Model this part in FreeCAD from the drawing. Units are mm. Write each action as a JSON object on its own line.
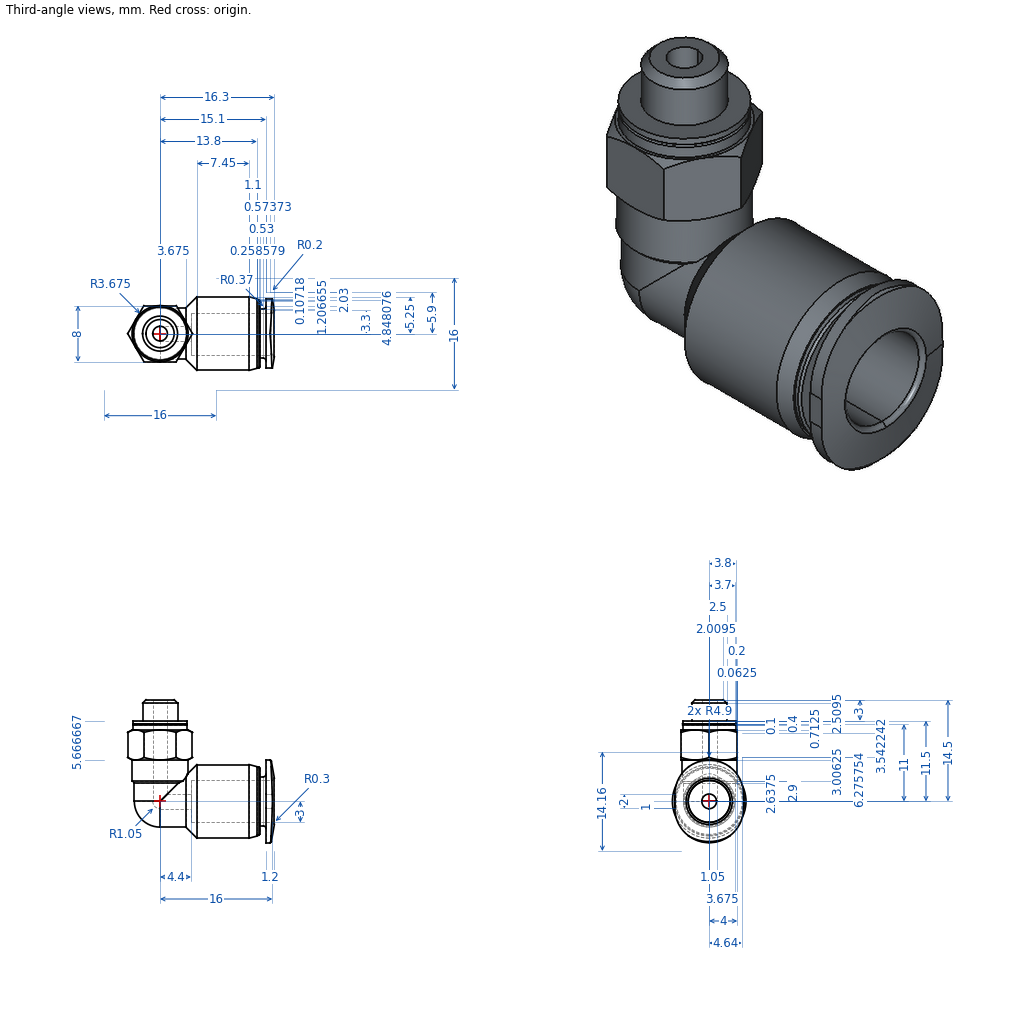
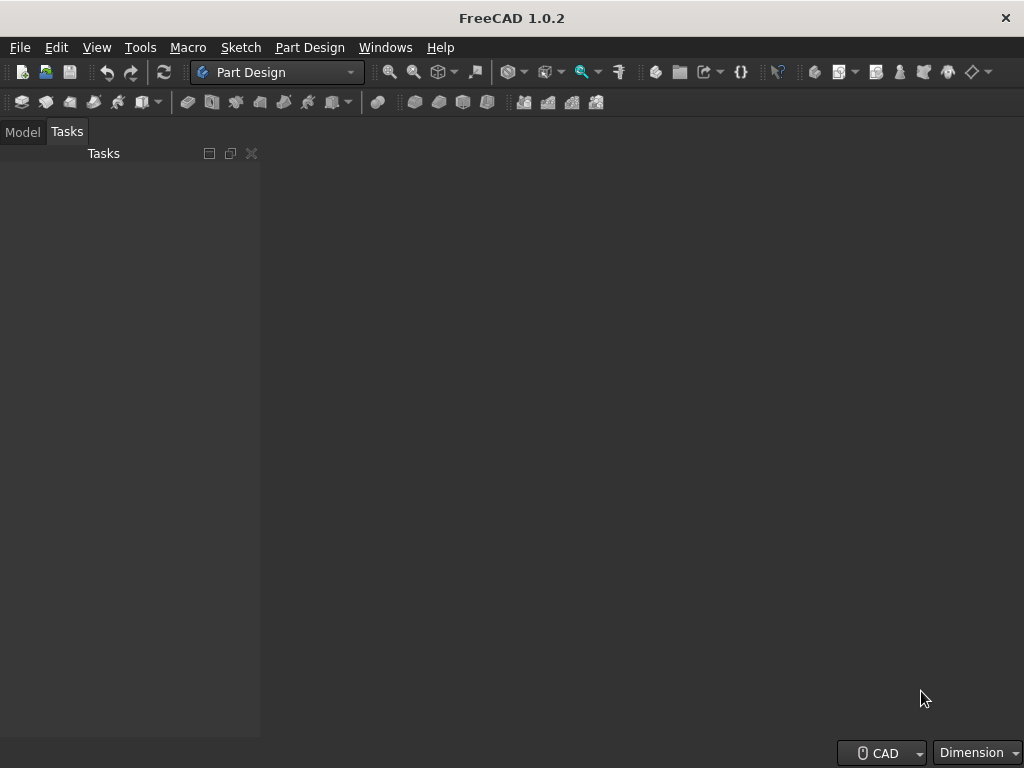
{"action": "left_click", "coordinate": [22, 72]}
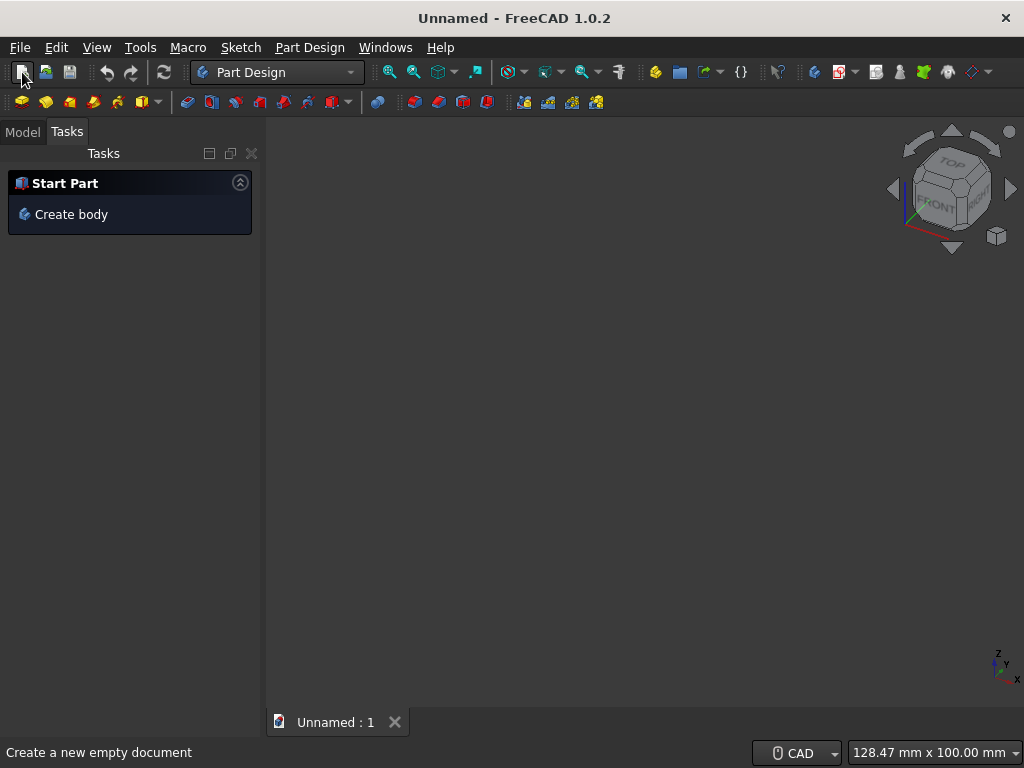
{"action": "left_click", "coordinate": [840, 72]}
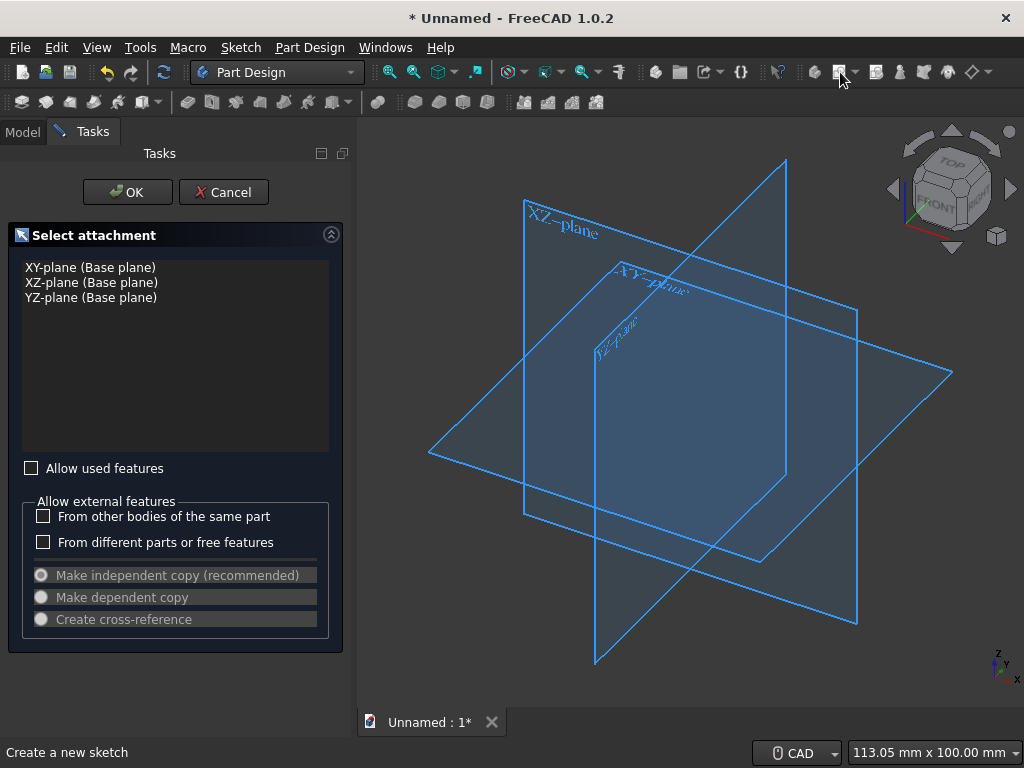
{"action": "left_click", "coordinate": [82, 268]}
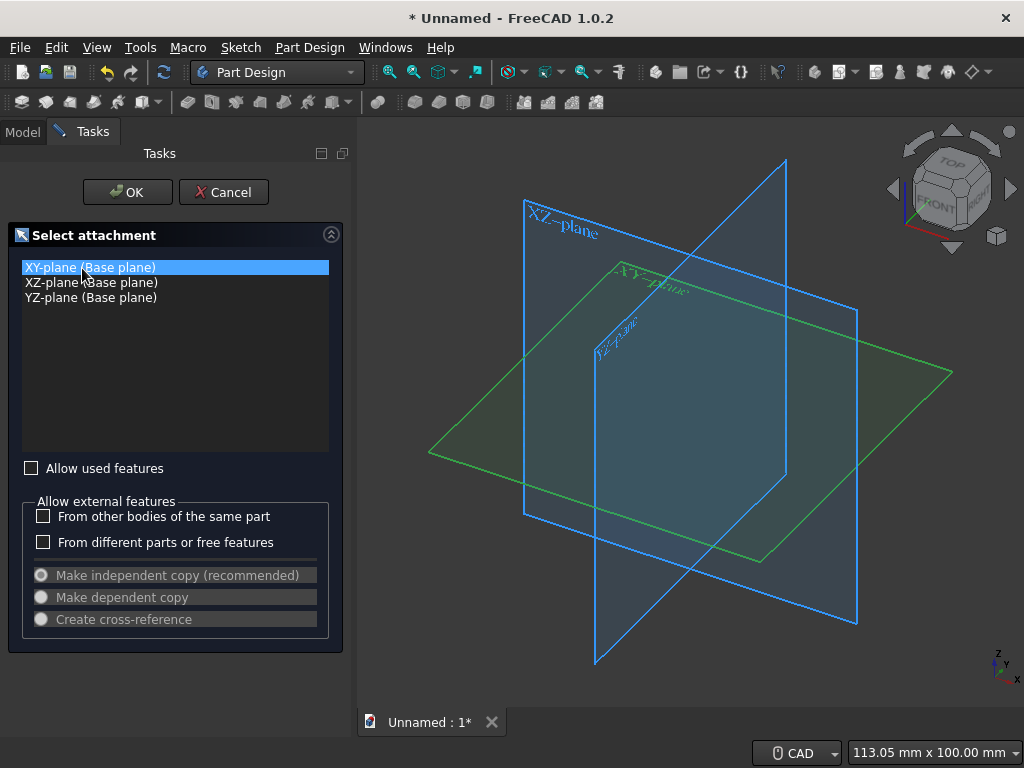
{"action": "left_click", "coordinate": [128, 192]}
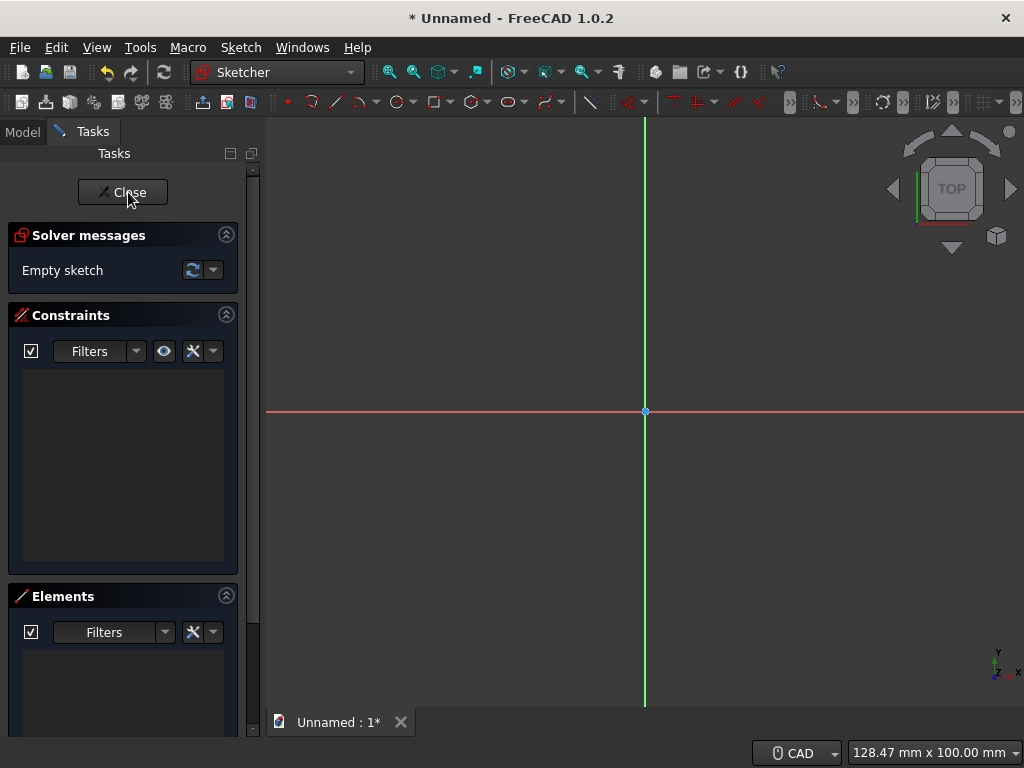
{"action": "scroll", "coordinate": [728, 387], "scroll_direction": "up", "scroll_amount": 6}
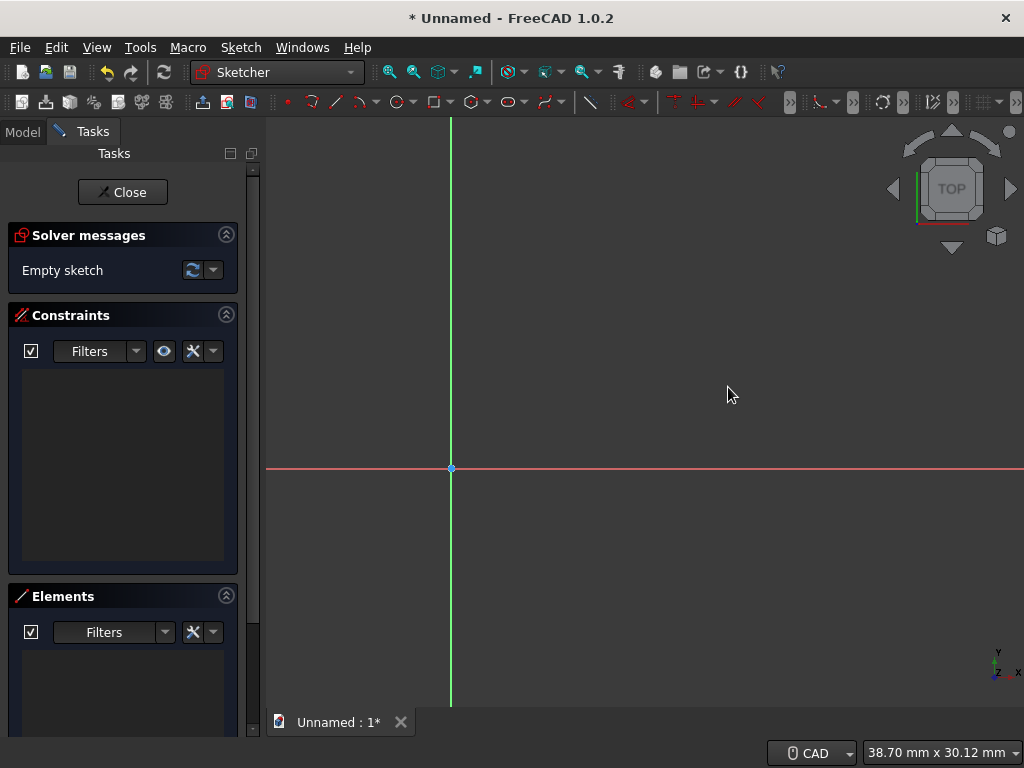
{"action": "left_click", "coordinate": [312, 102]}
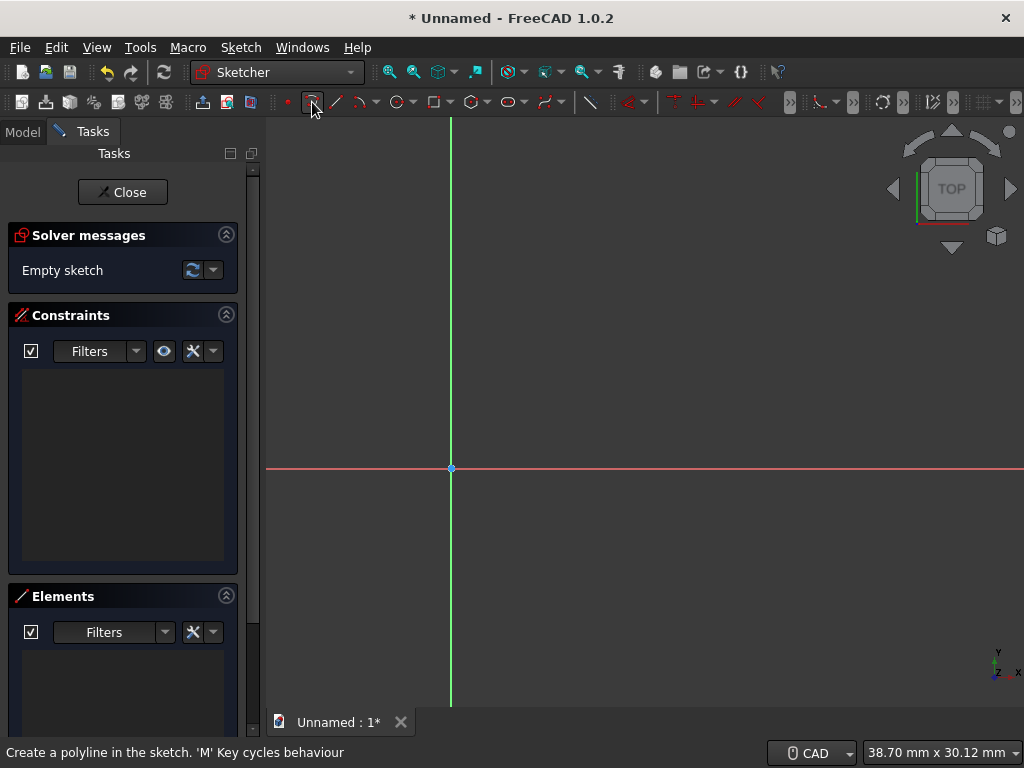
{"action": "left_click", "coordinate": [379, 469]}
{"action": "left_click", "coordinate": [770, 460]}
{"action": "left_click", "coordinate": [770, 404]}
{"action": "left_click", "coordinate": [762, 357]}
{"action": "right_click", "coordinate": [762, 357]}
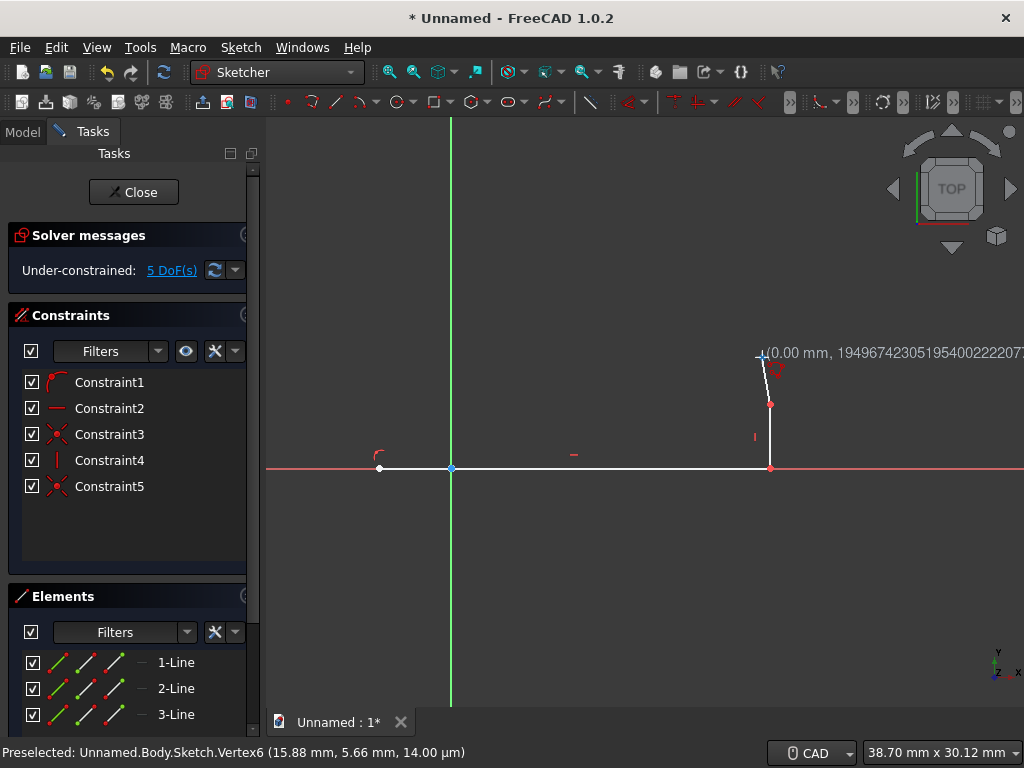
{"action": "scroll", "coordinate": [758, 353], "scroll_direction": "up", "scroll_amount": 6}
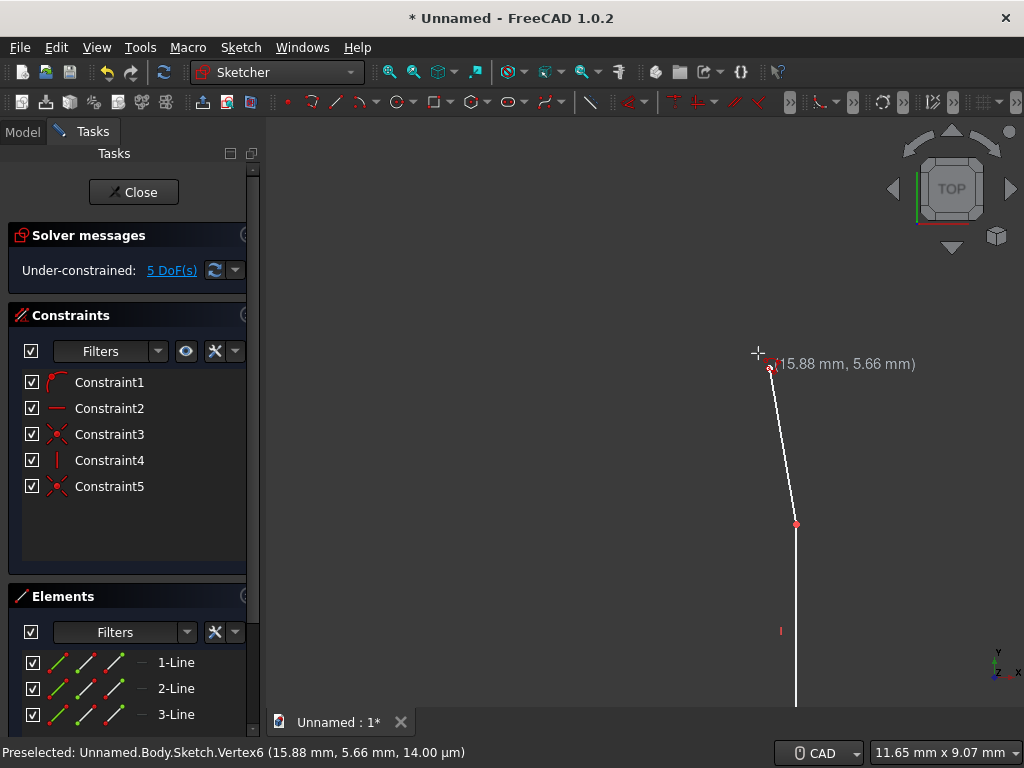
{"action": "left_click", "coordinate": [757, 353]}
{"action": "left_click", "coordinate": [719, 353]}
{"action": "left_click", "coordinate": [719, 485]}
{"action": "right_click", "coordinate": [719, 485]}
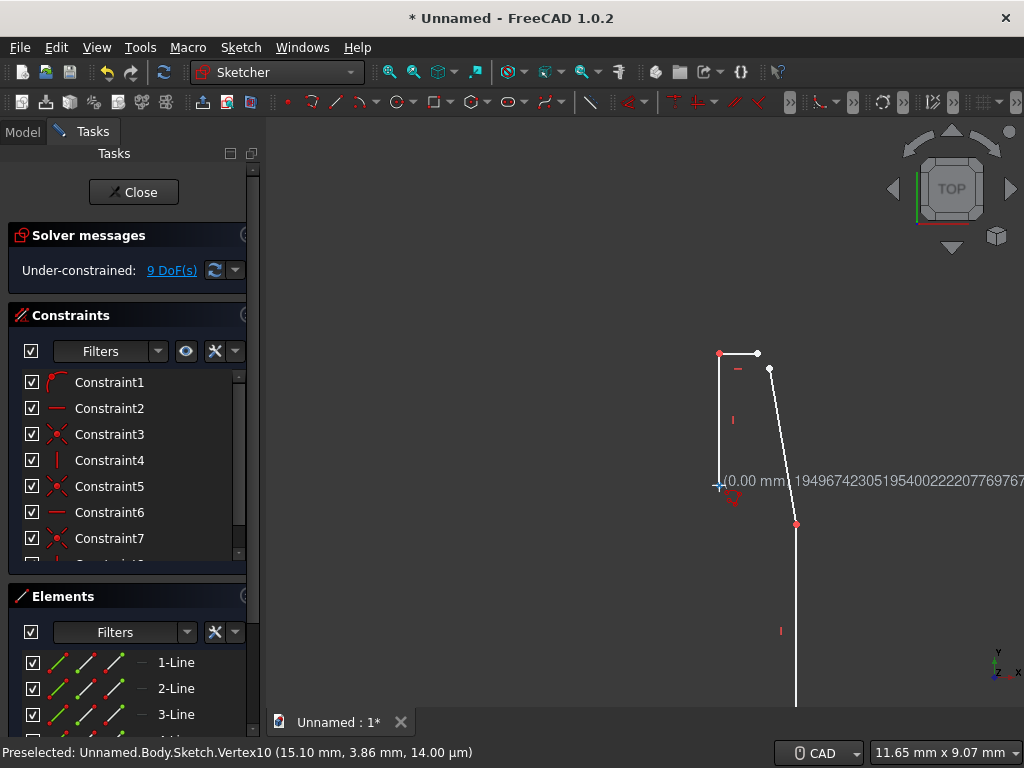
{"action": "left_click", "coordinate": [695, 509]}
{"action": "left_click", "coordinate": [661, 509]}
{"action": "left_click", "coordinate": [661, 431]}
{"action": "left_click", "coordinate": [652, 422]}
{"action": "left_click", "coordinate": [635, 422]}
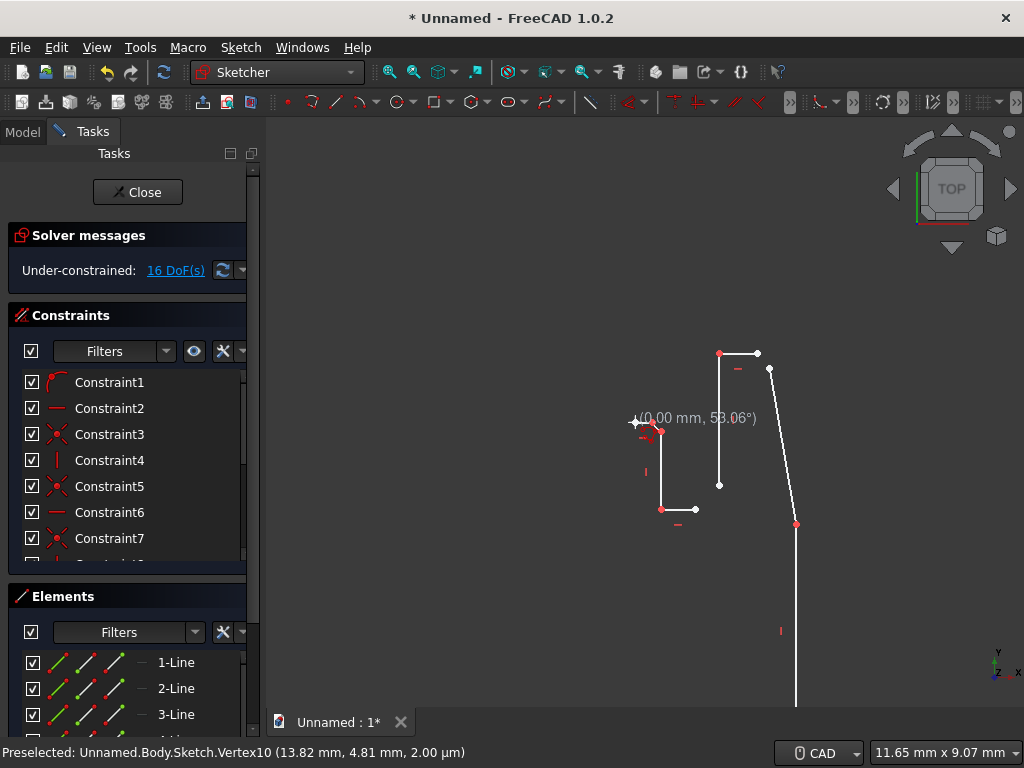
{"action": "scroll", "coordinate": [635, 415], "scroll_direction": "up", "scroll_amount": 5}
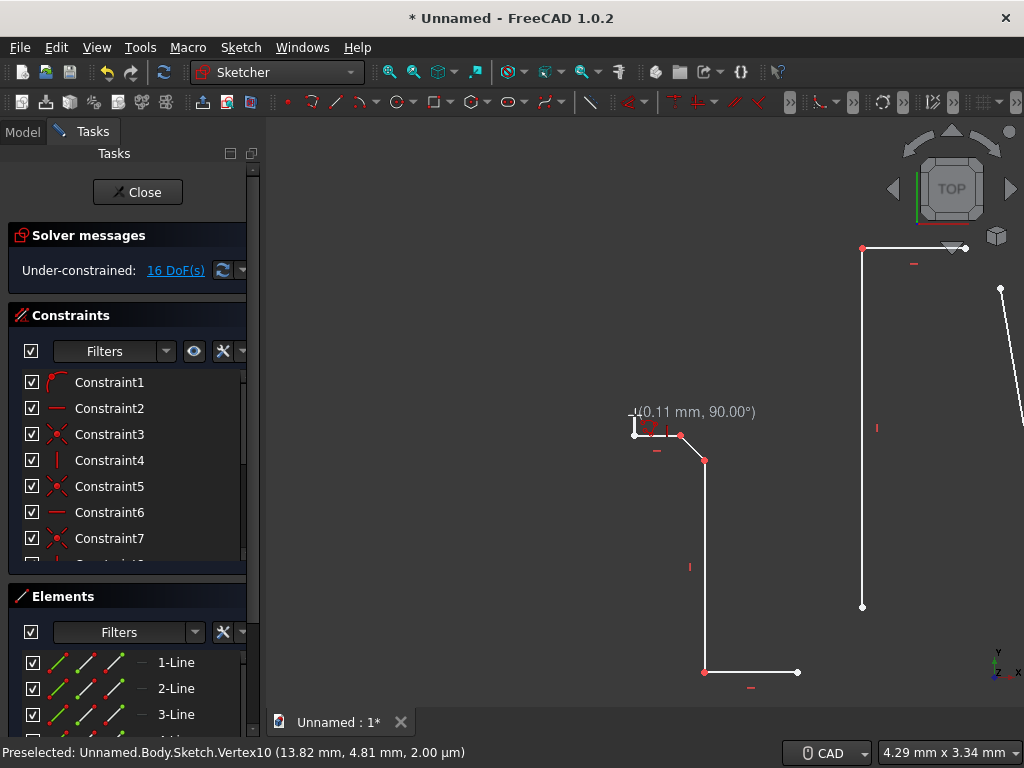
{"action": "left_click", "coordinate": [634, 413]}